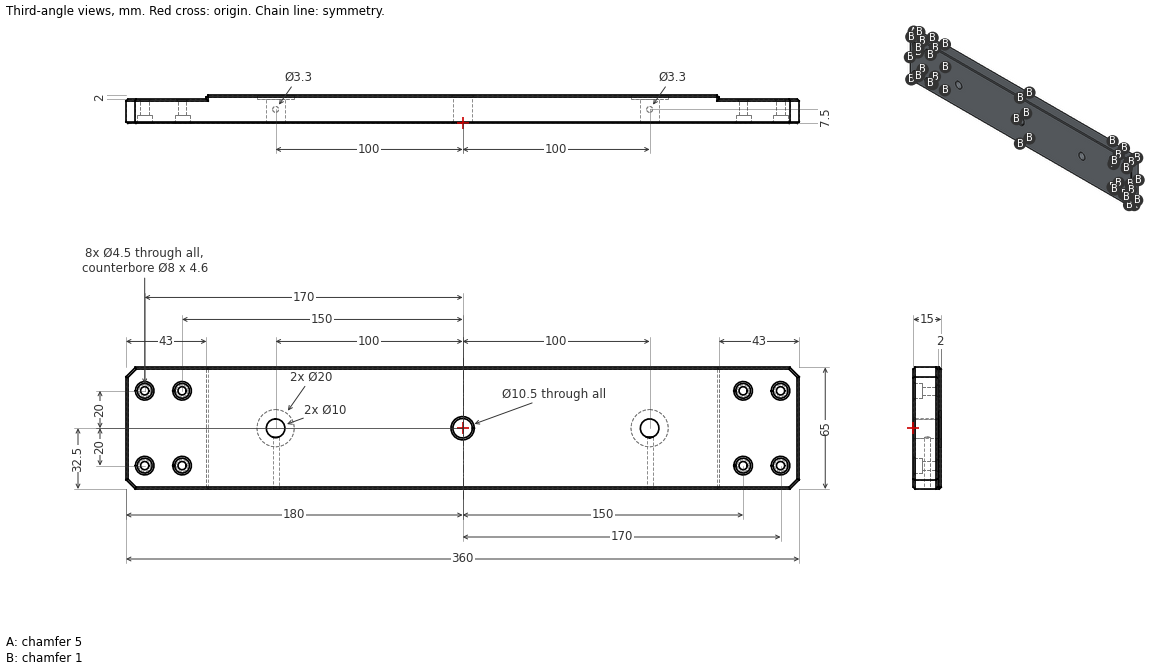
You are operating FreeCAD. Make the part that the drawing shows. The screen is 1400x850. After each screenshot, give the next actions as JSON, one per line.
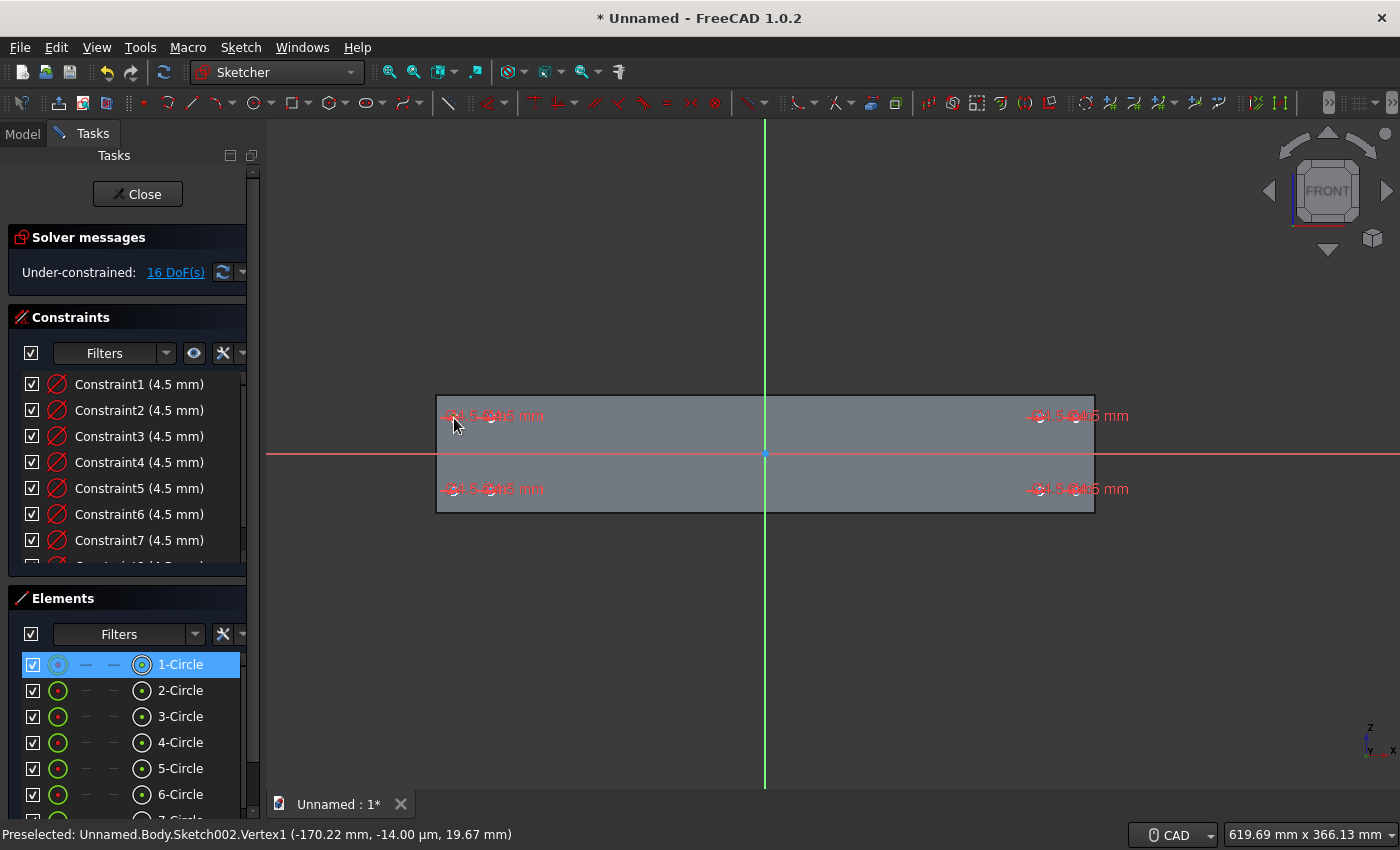
{"action": "left_click", "coordinate": [491, 418]}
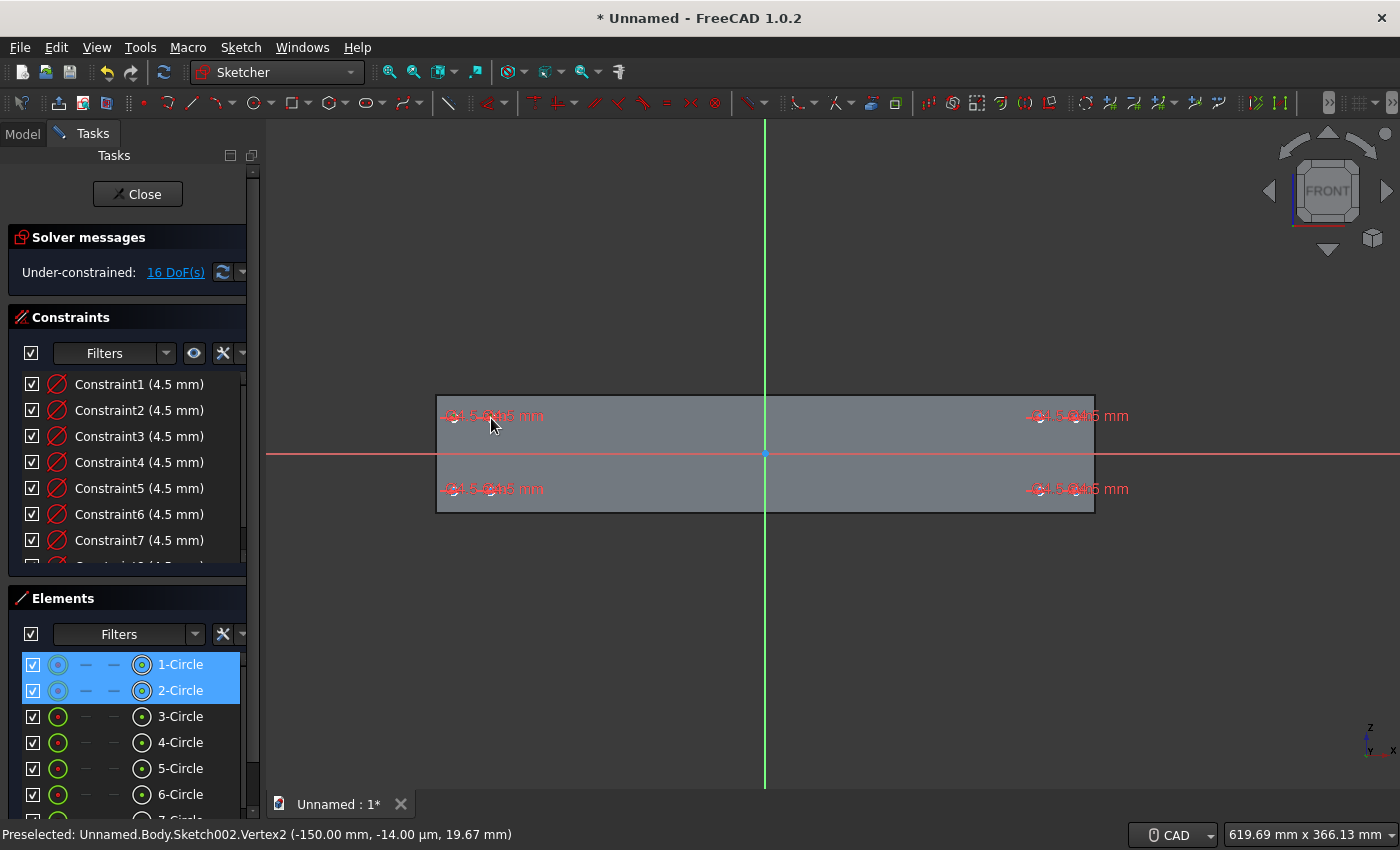
{"action": "left_click", "coordinate": [576, 104]}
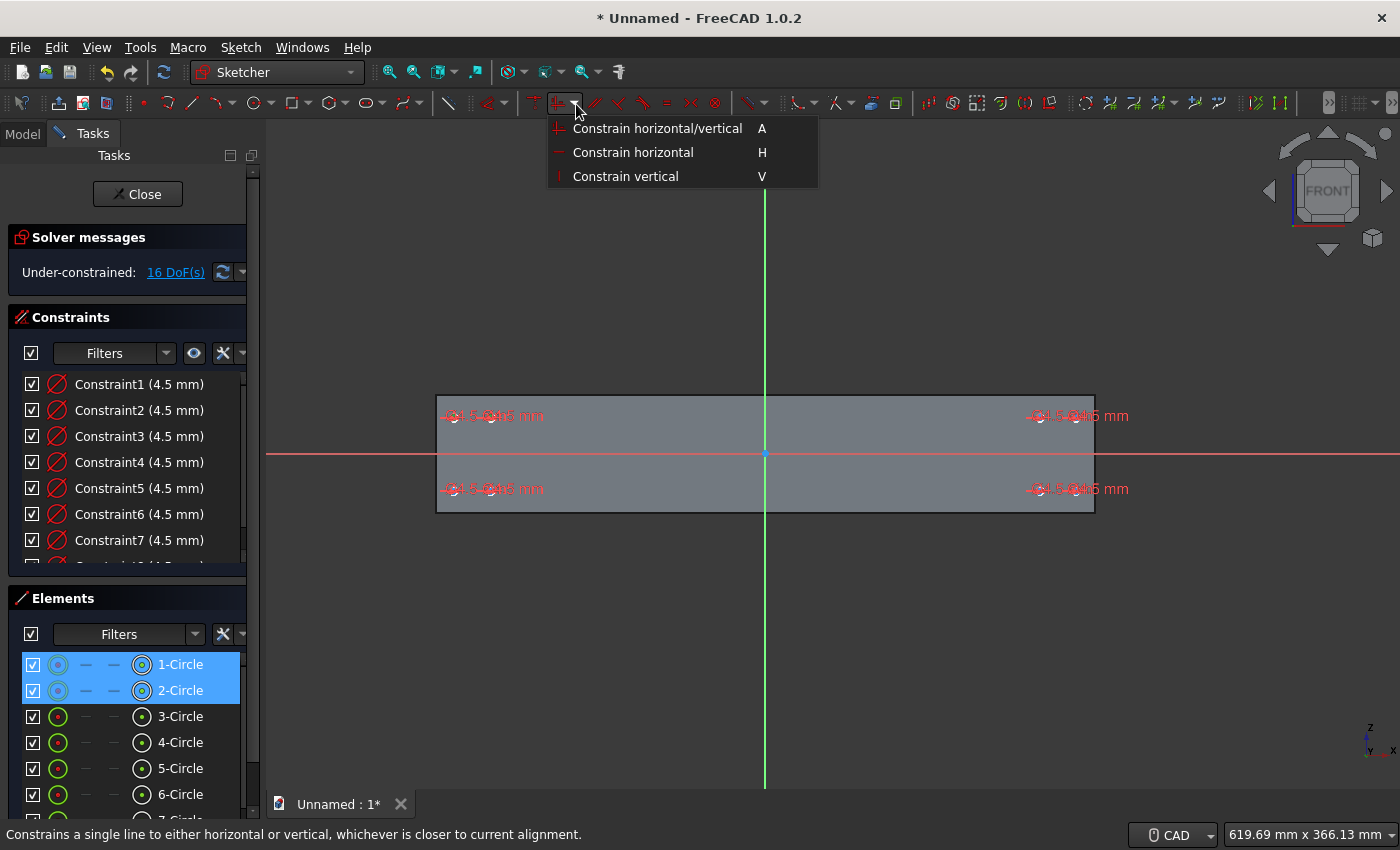
{"action": "left_click", "coordinate": [683, 152]}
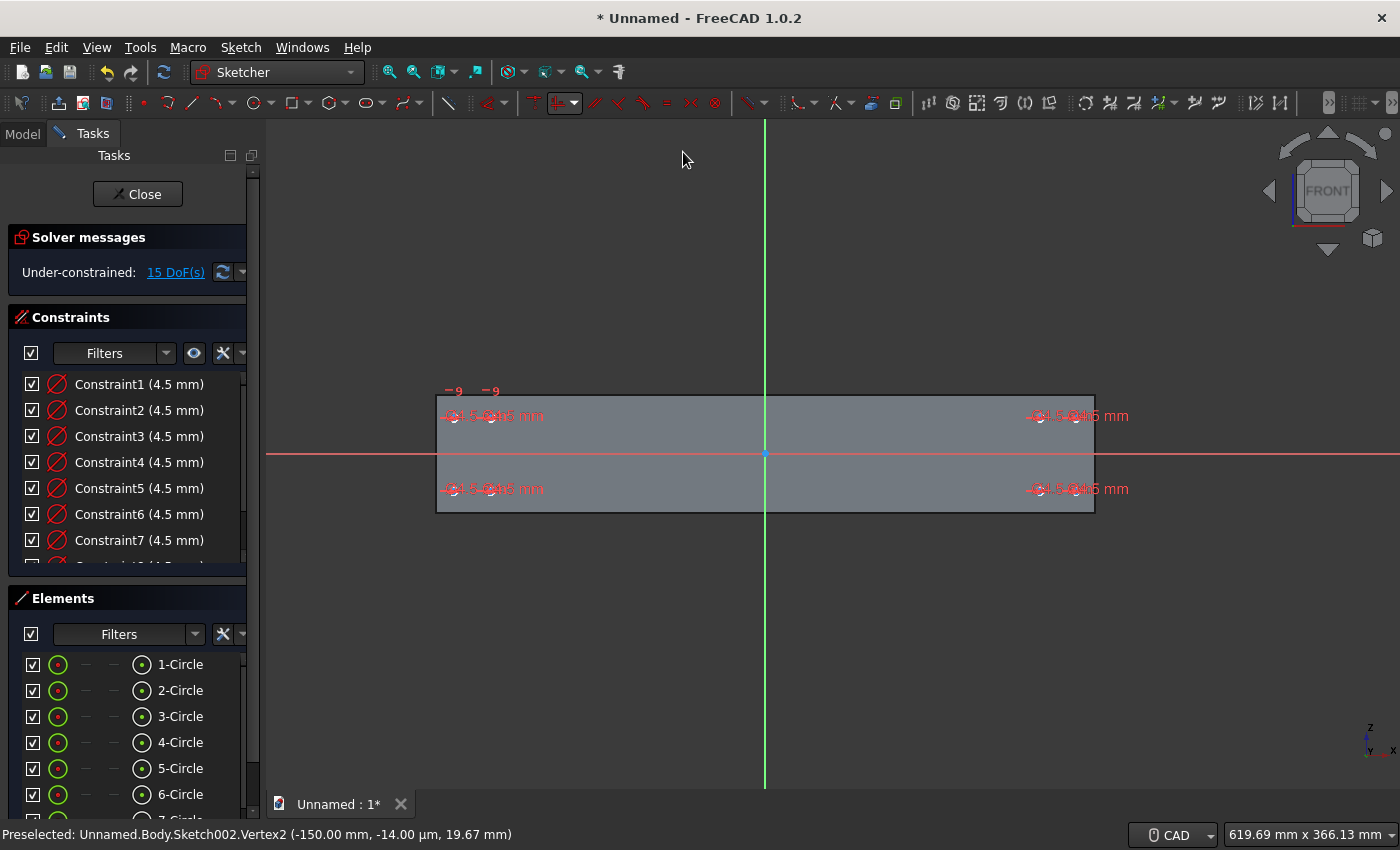
{"action": "left_click", "coordinate": [454, 418]}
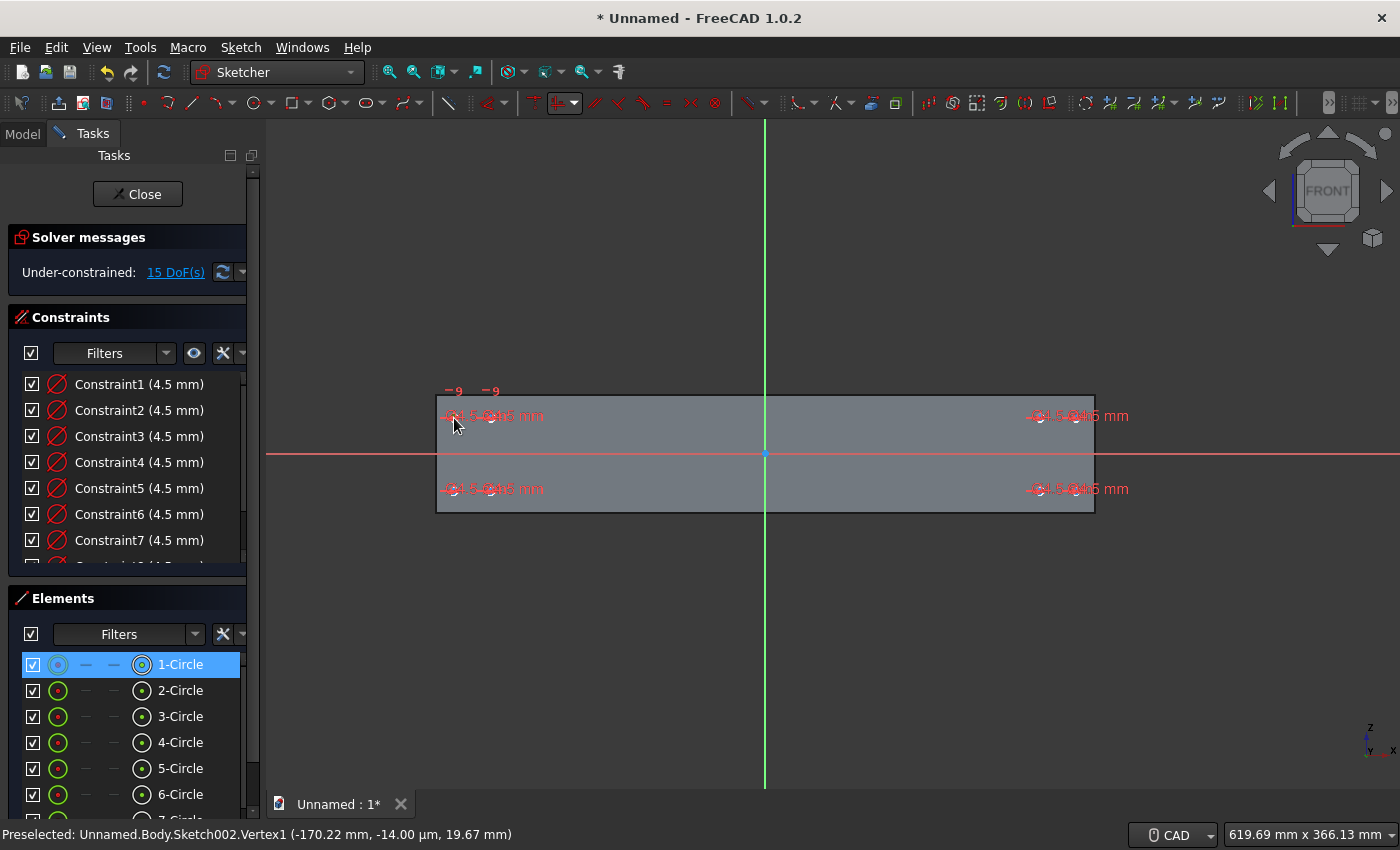
{"action": "left_click", "coordinate": [454, 491]}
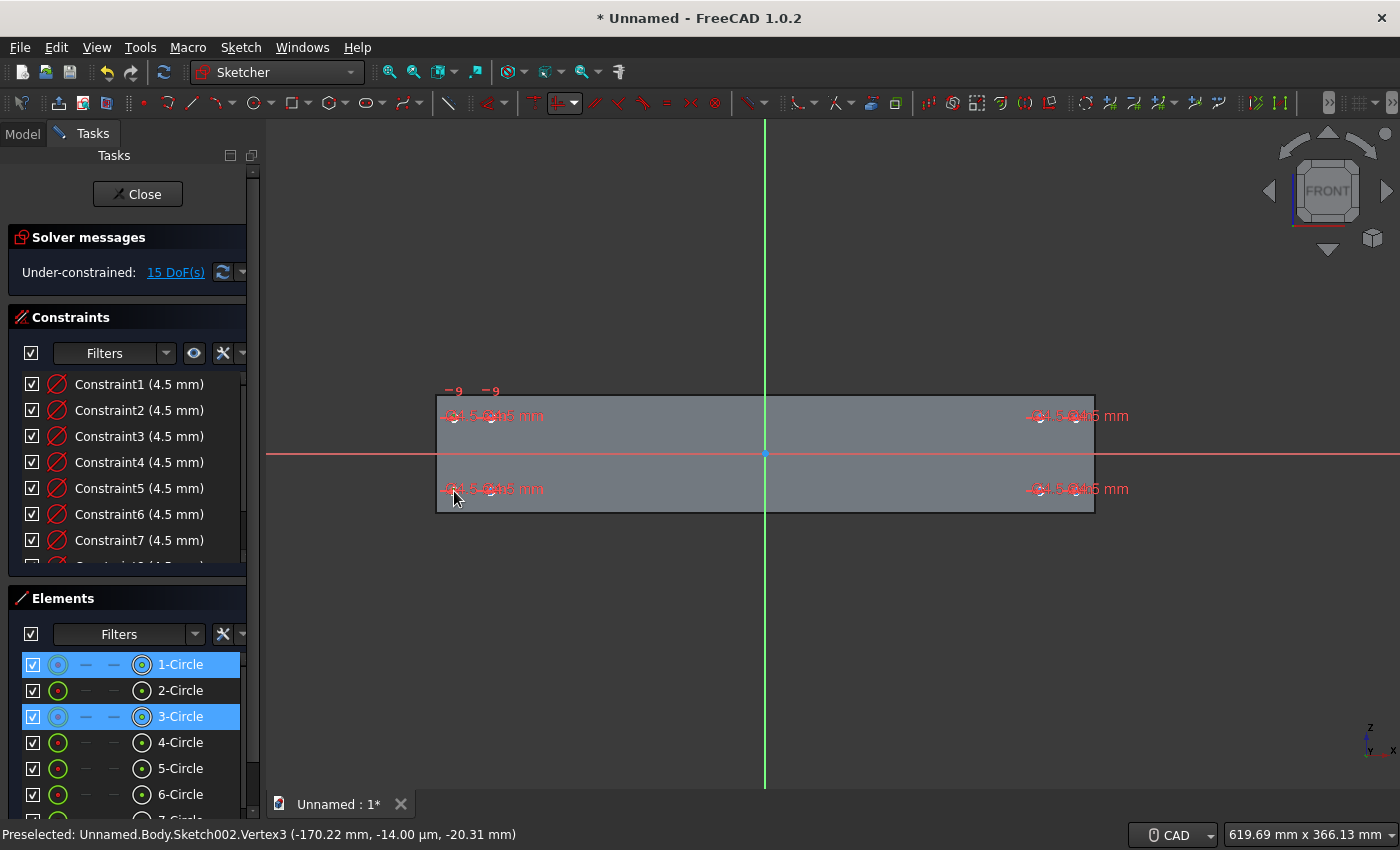
{"action": "left_click", "coordinate": [576, 104]}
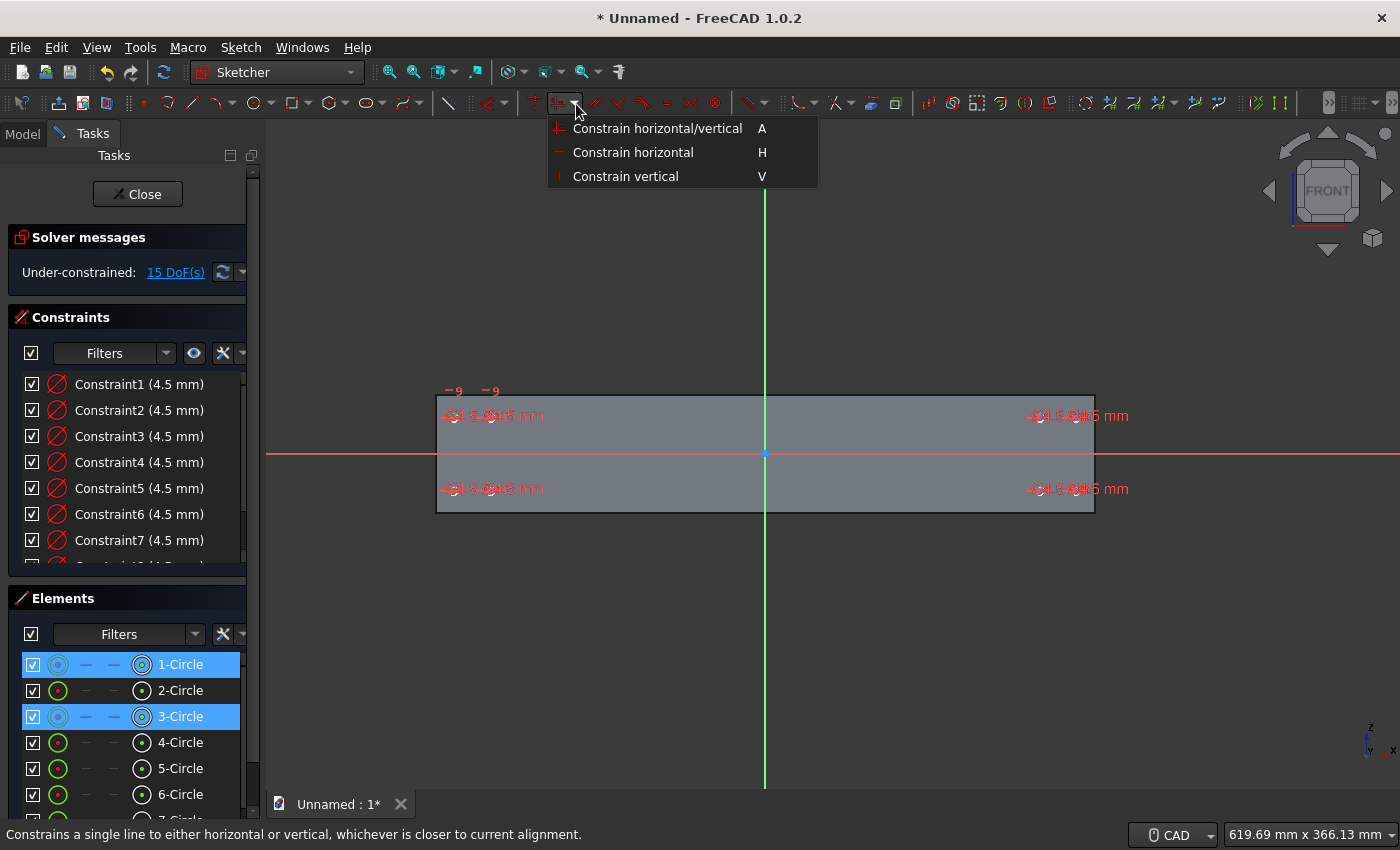
{"action": "left_click", "coordinate": [683, 176]}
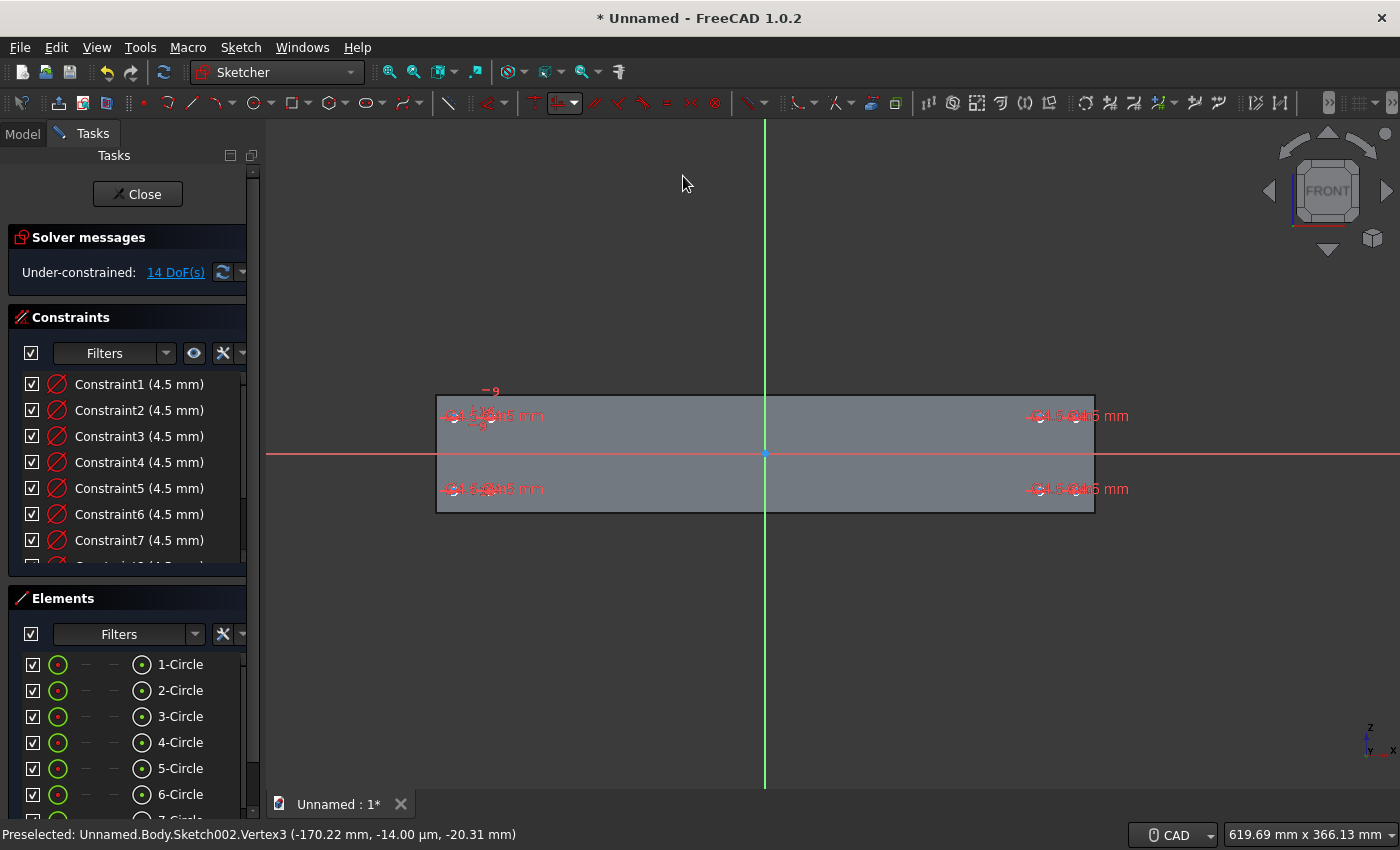
{"action": "left_click", "coordinate": [491, 418]}